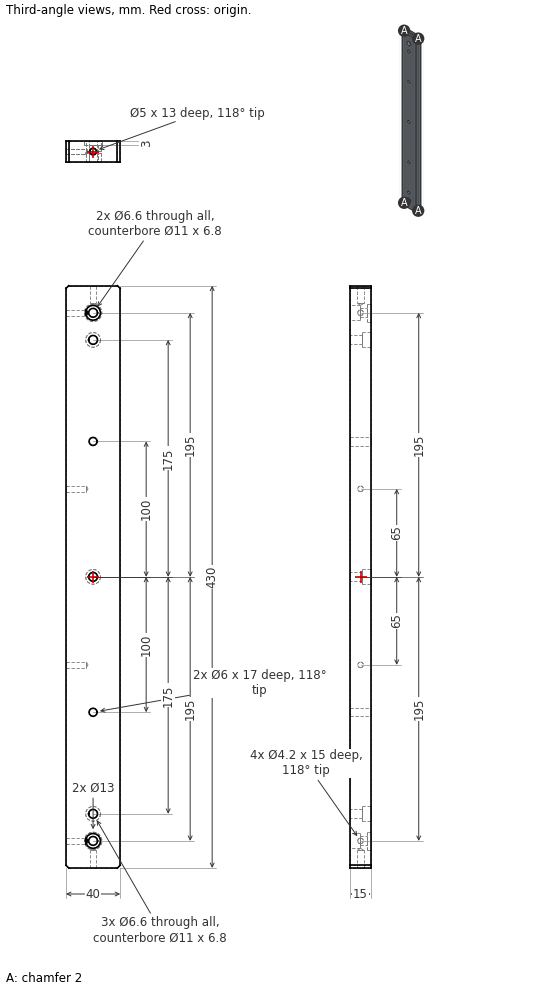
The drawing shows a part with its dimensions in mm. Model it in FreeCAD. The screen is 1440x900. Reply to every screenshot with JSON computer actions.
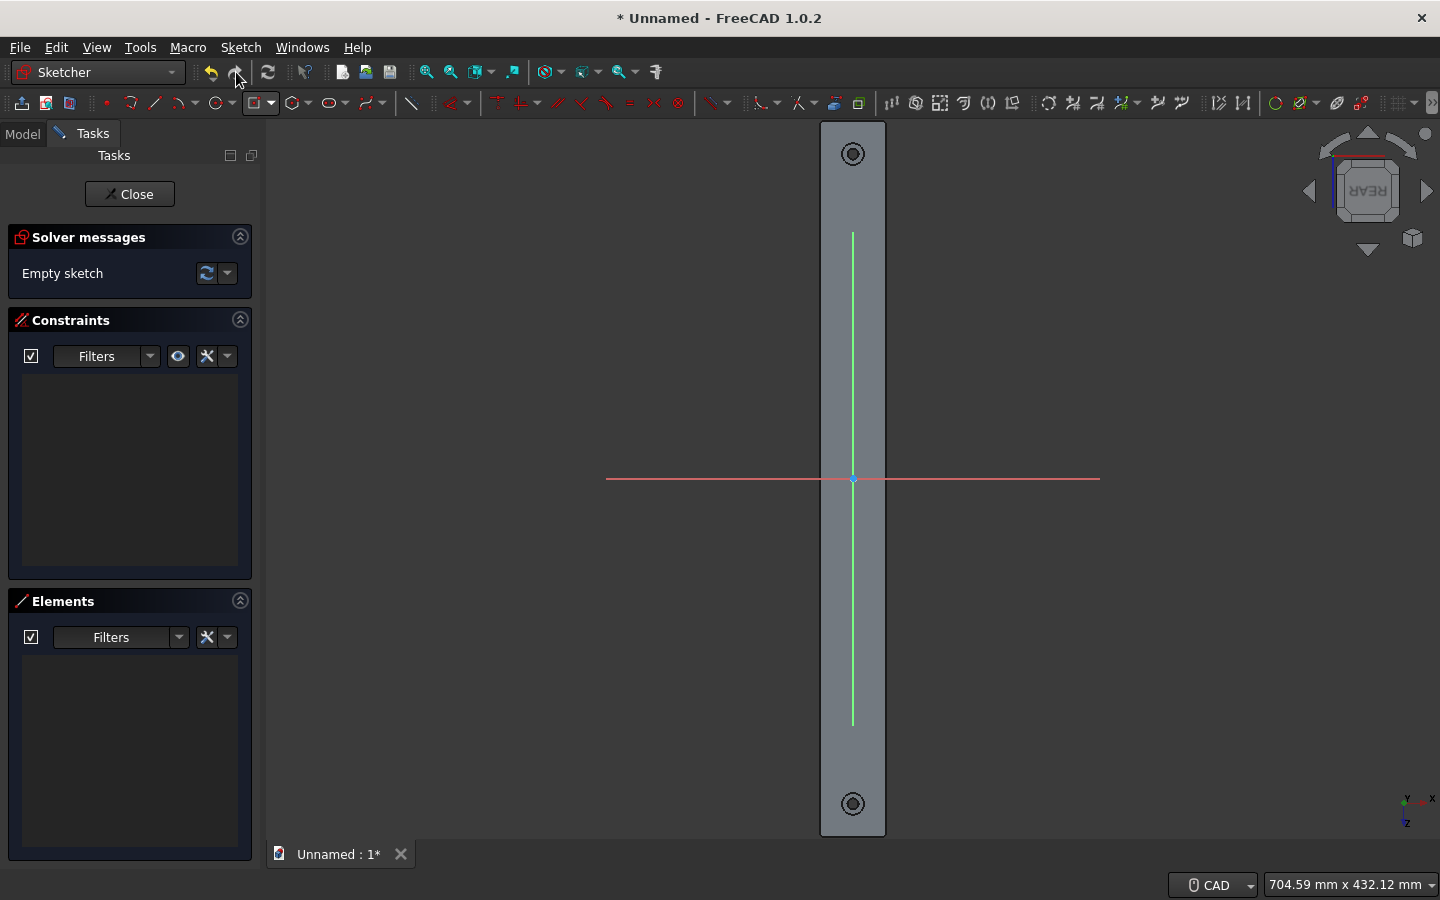
{"action": "key", "text": "g c"}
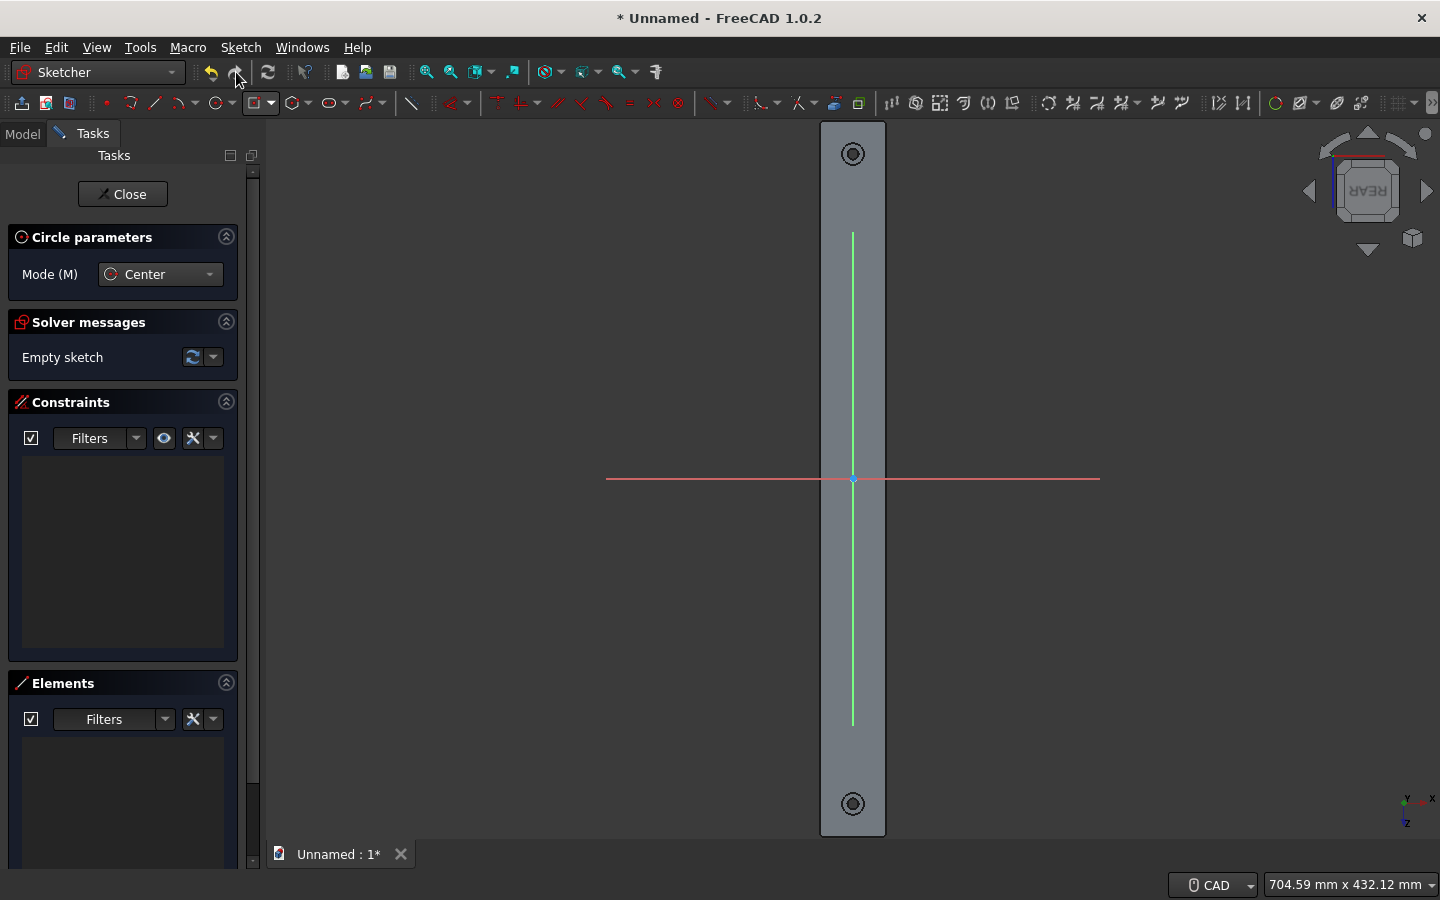
{"action": "scroll", "coordinate": [853, 187], "scroll_direction": "up", "scroll_amount": 8}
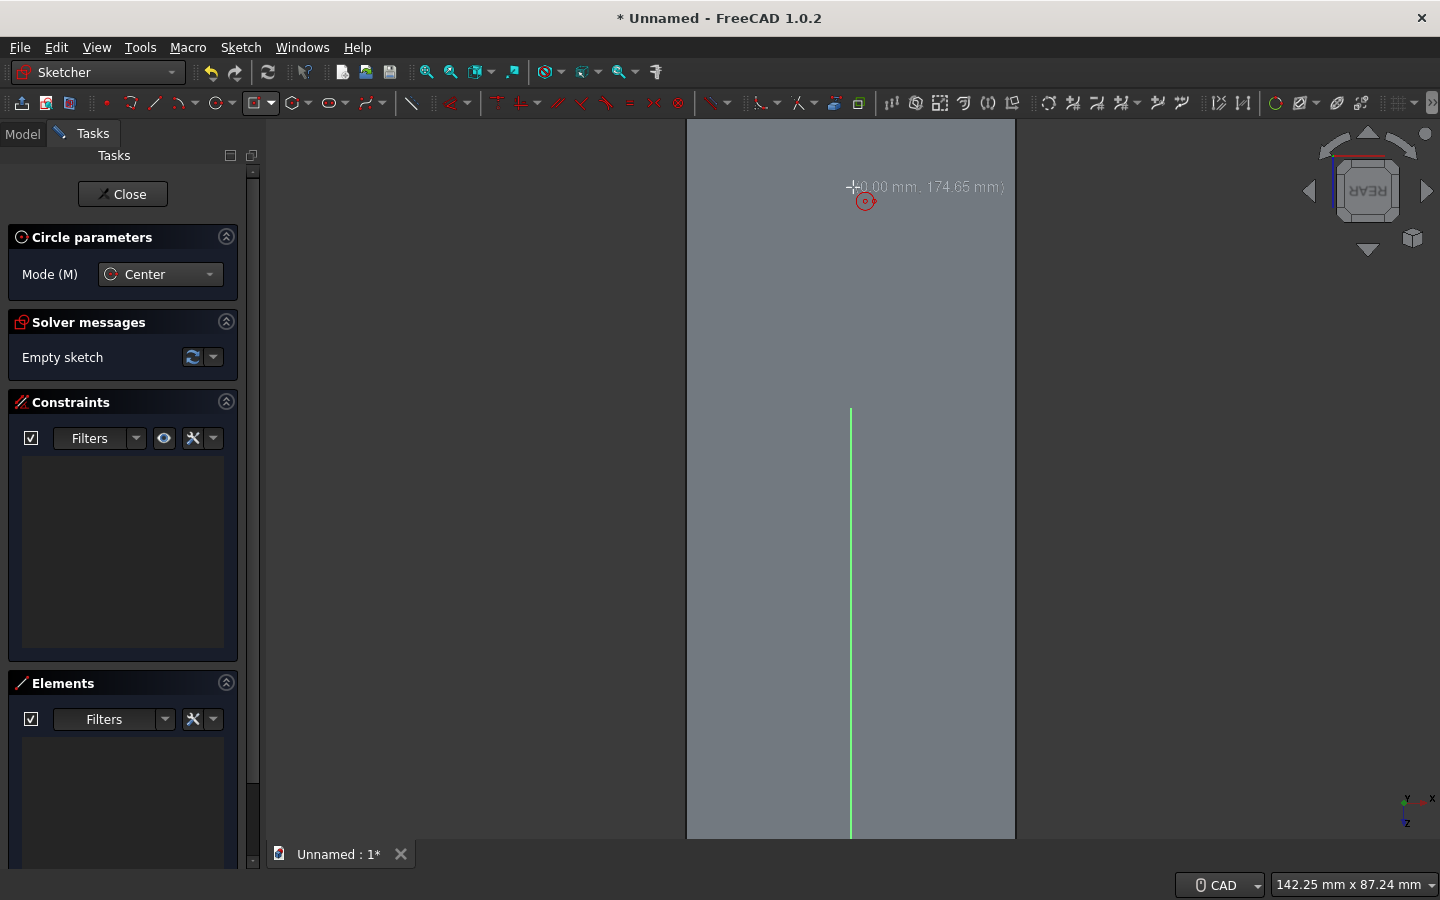
{"action": "scroll", "coordinate": [771, 250], "scroll_direction": "down", "scroll_amount": 9}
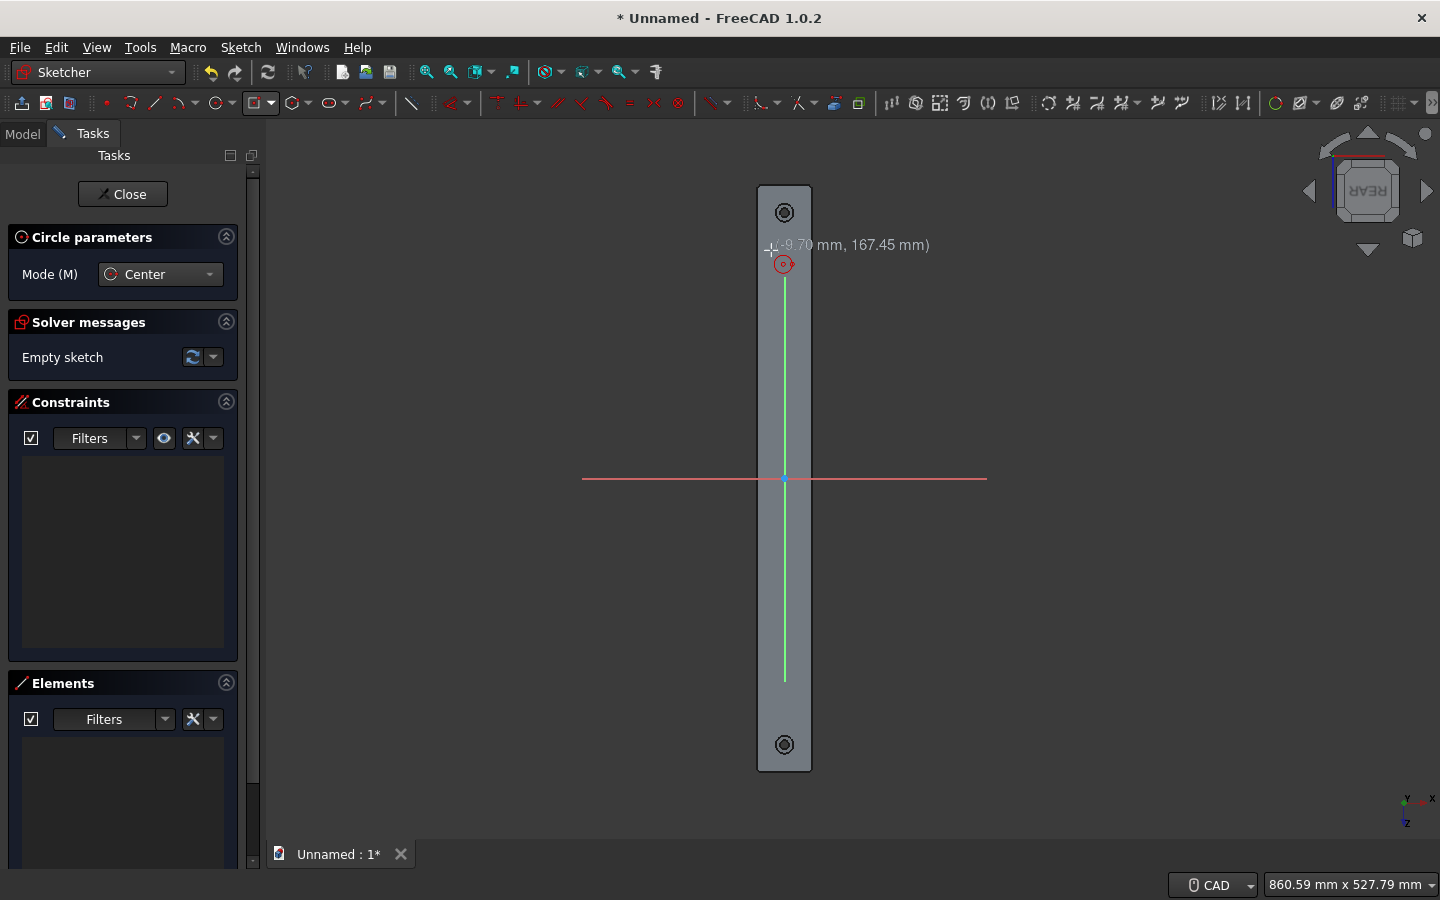
{"action": "left_click", "coordinate": [785, 240]}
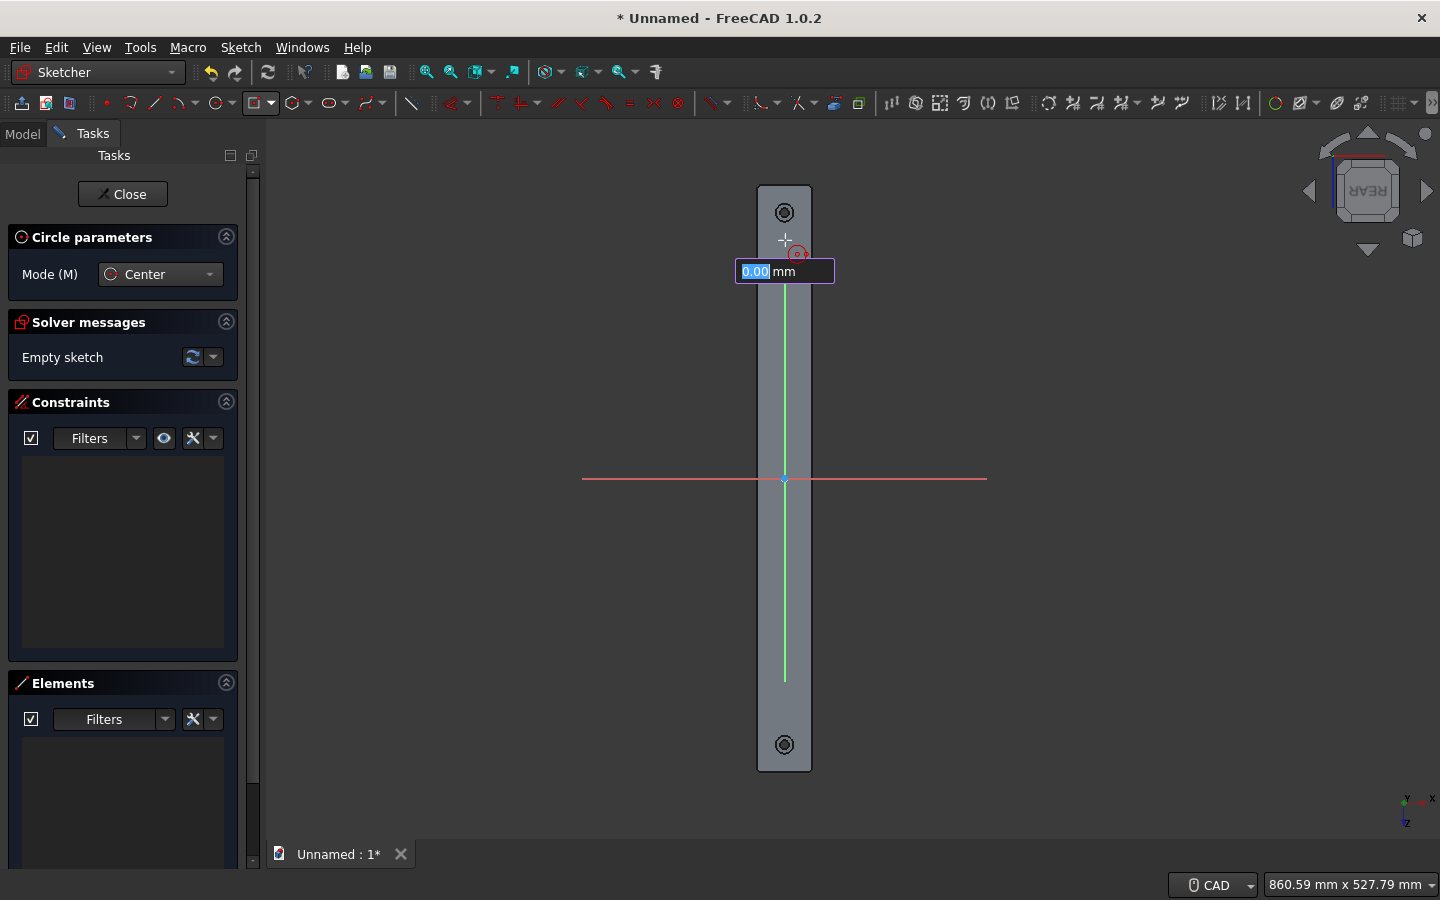
{"action": "scroll", "coordinate": [789, 238], "scroll_direction": "up", "scroll_amount": 7}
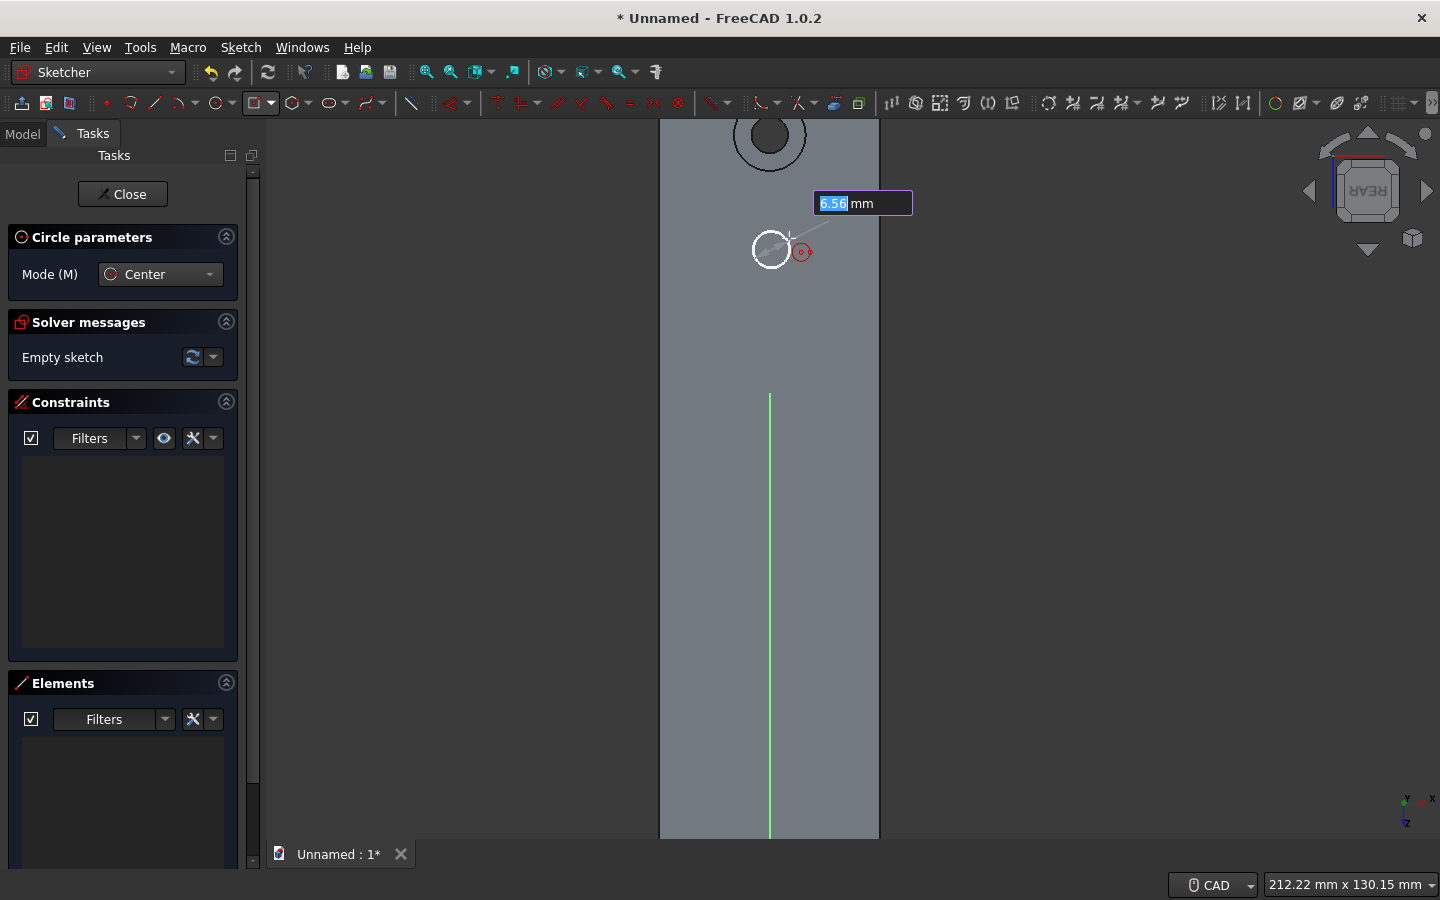
{"action": "left_click", "coordinate": [787, 239]}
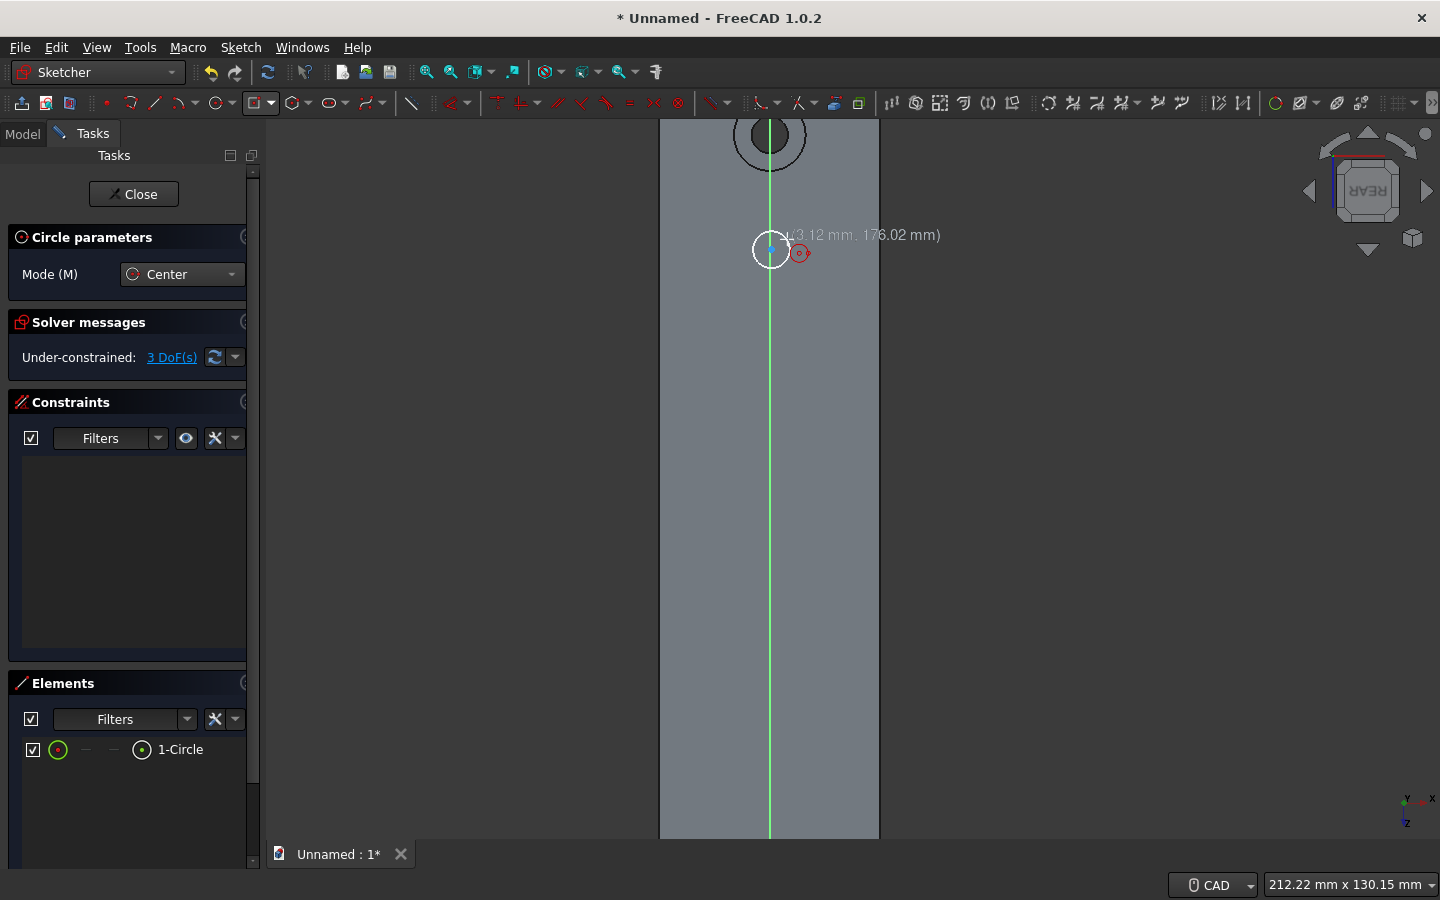
{"action": "scroll", "coordinate": [789, 239], "scroll_direction": "down", "scroll_amount": 7}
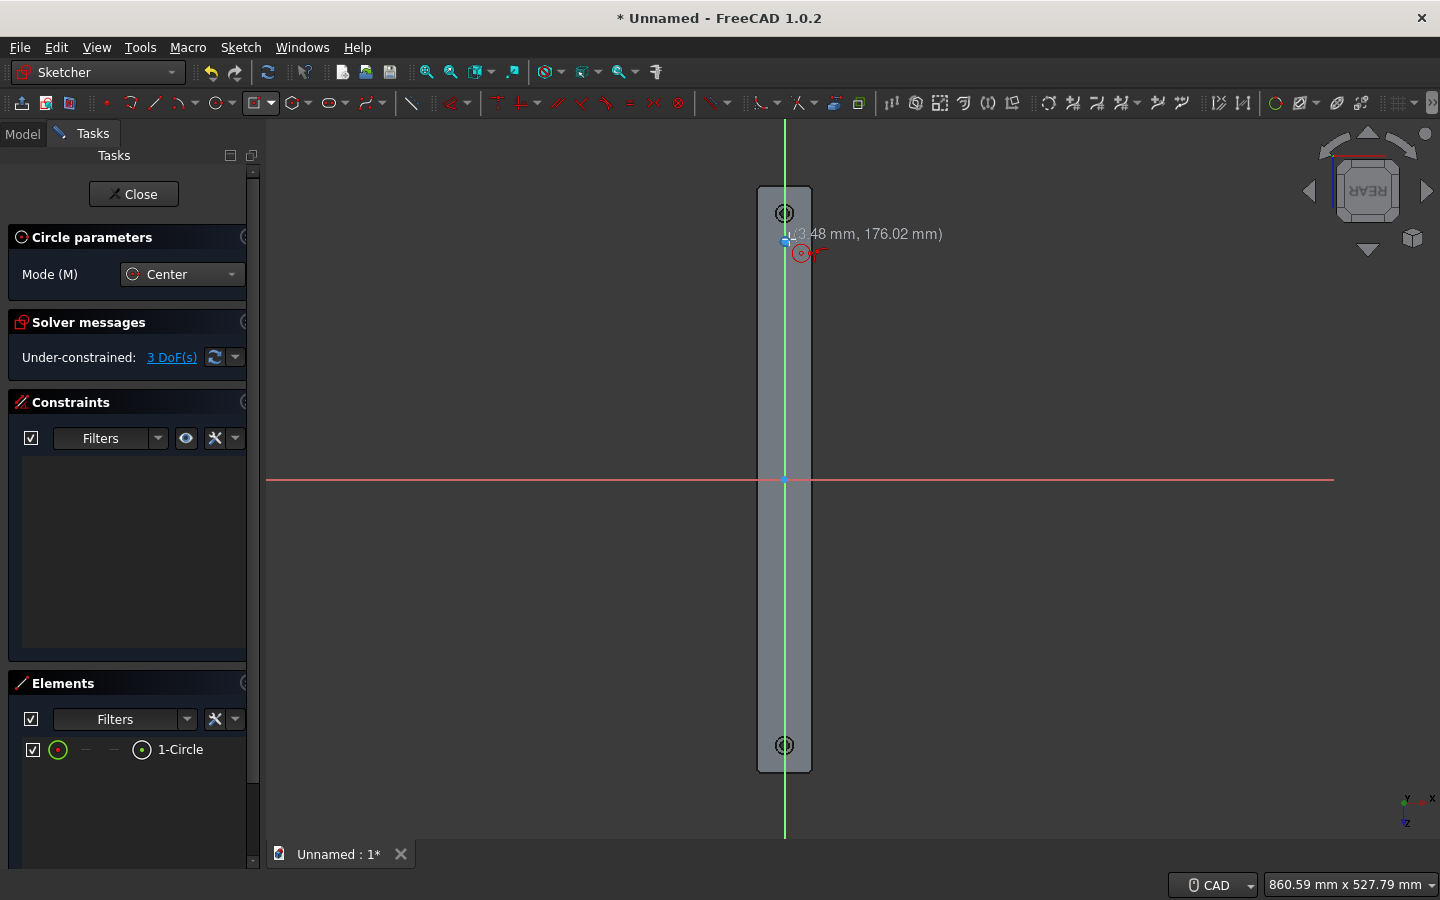
{"action": "scroll", "coordinate": [785, 718], "scroll_direction": "up", "scroll_amount": 9}